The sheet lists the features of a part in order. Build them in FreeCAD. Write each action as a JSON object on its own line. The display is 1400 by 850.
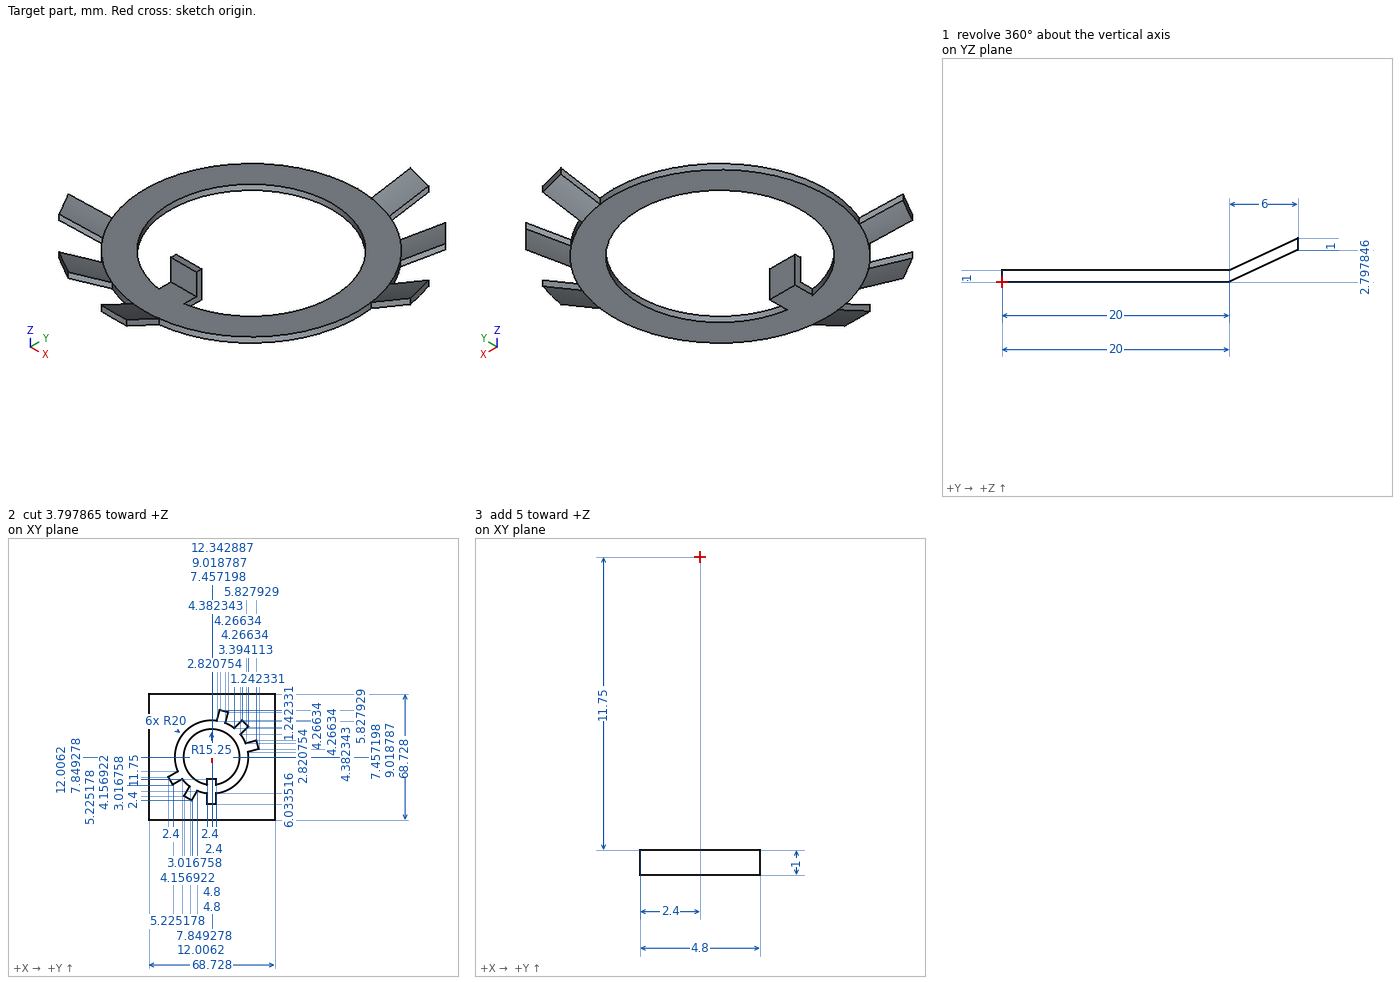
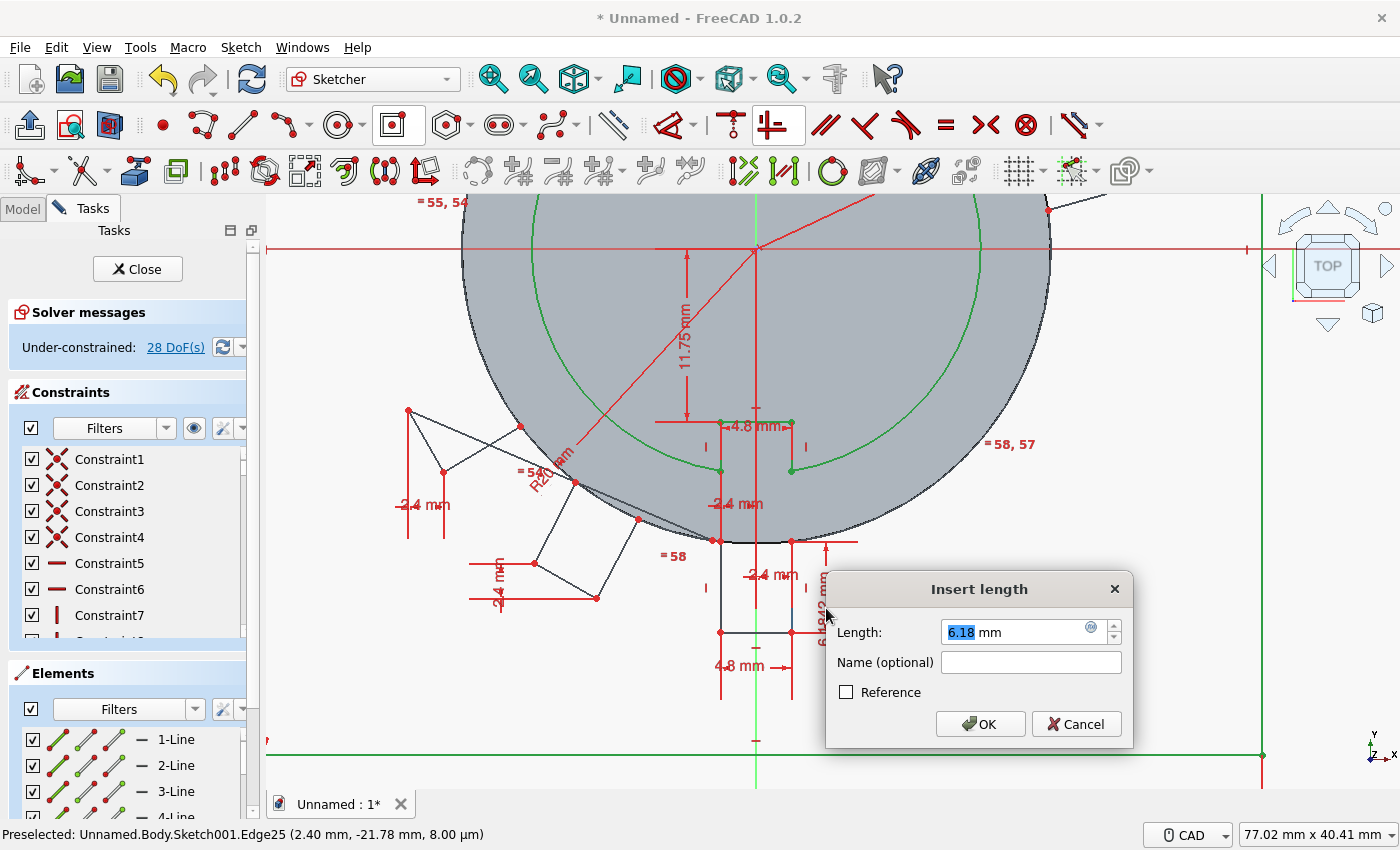
{"action": "type", "text": "6.033516"}
{"action": "key", "text": "Return"}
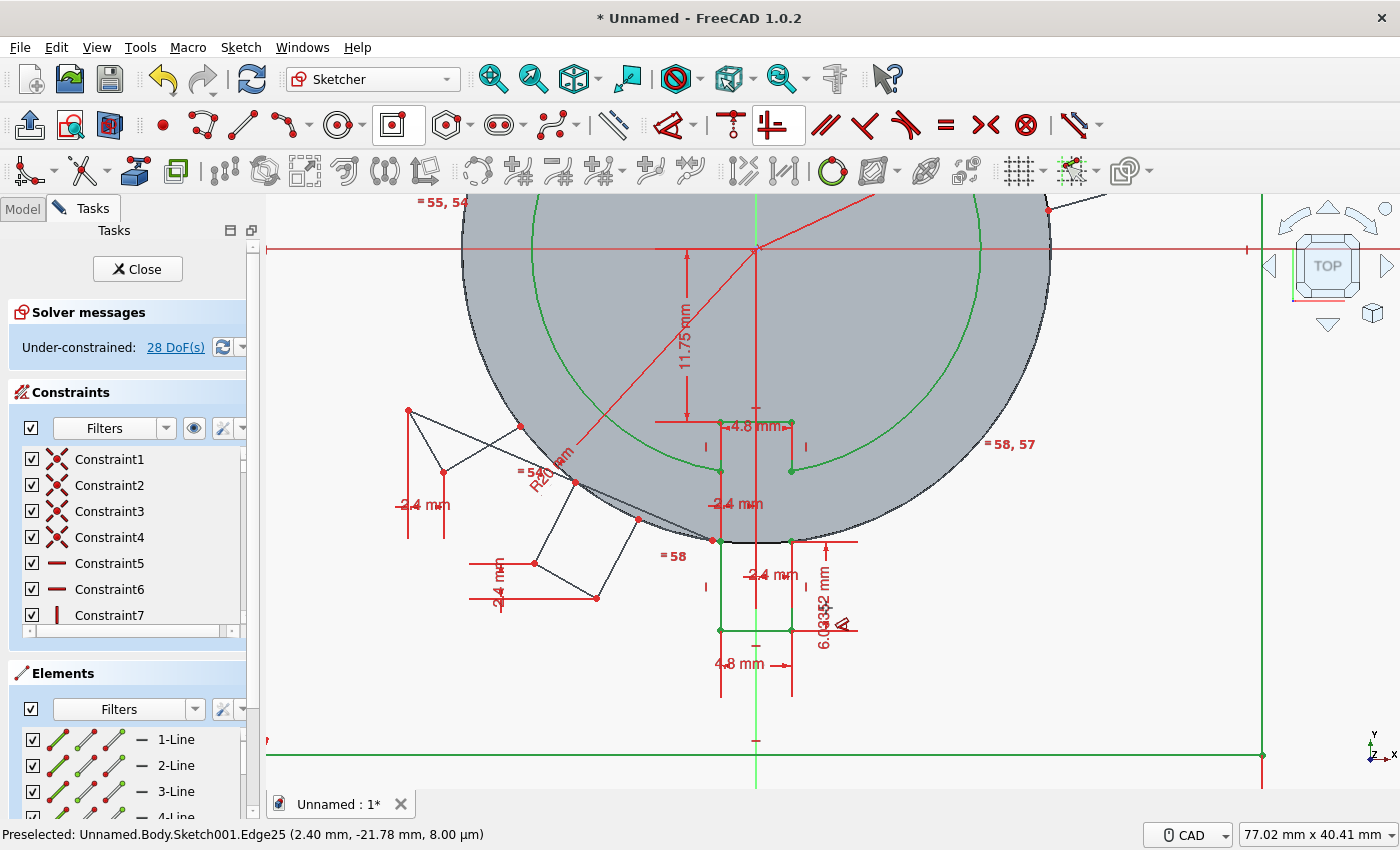
{"action": "left_click", "coordinate": [576, 482]}
{"action": "left_click", "coordinate": [603, 516]}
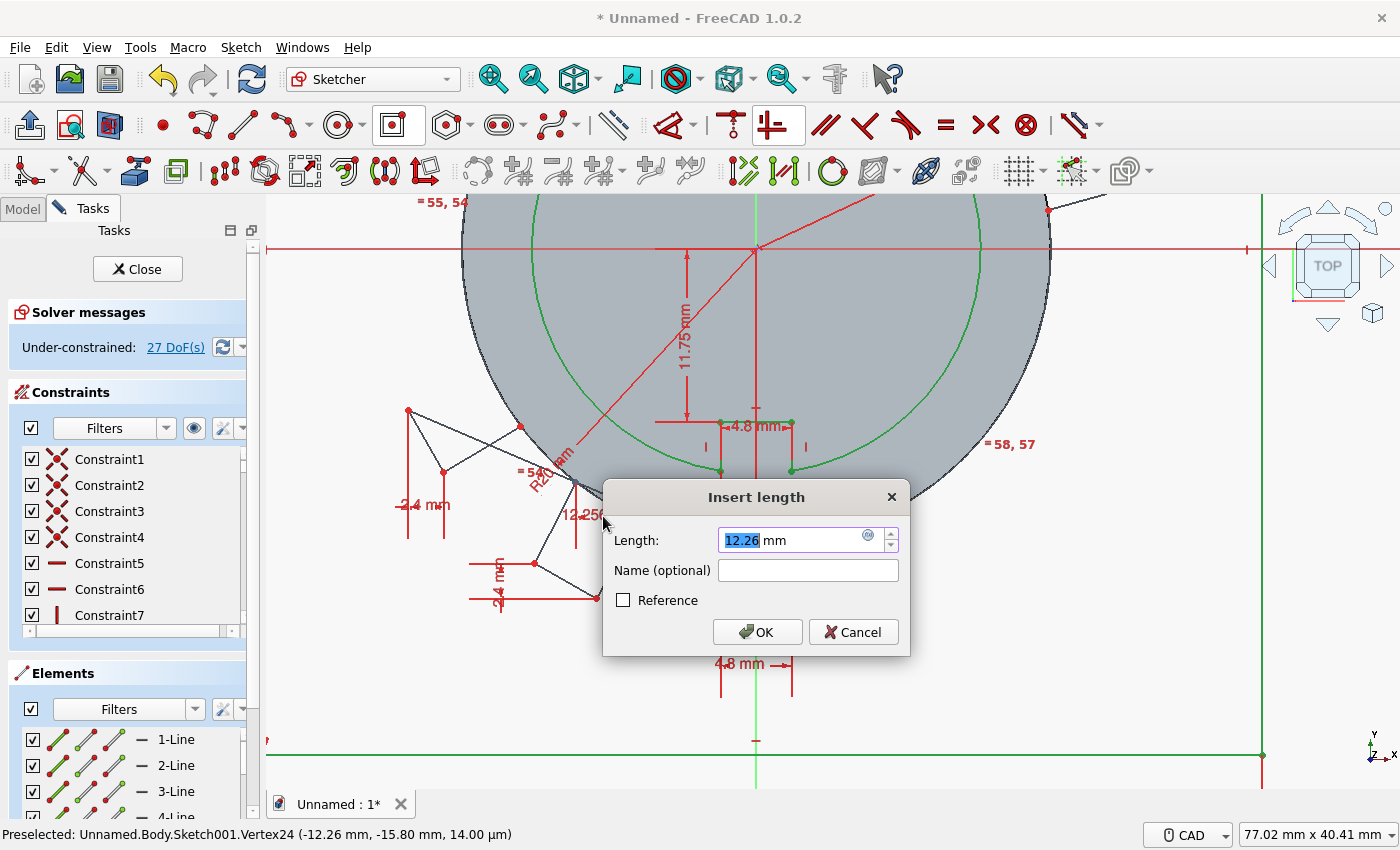
{"action": "type", "text": "12.0062"}
{"action": "key", "text": "Return"}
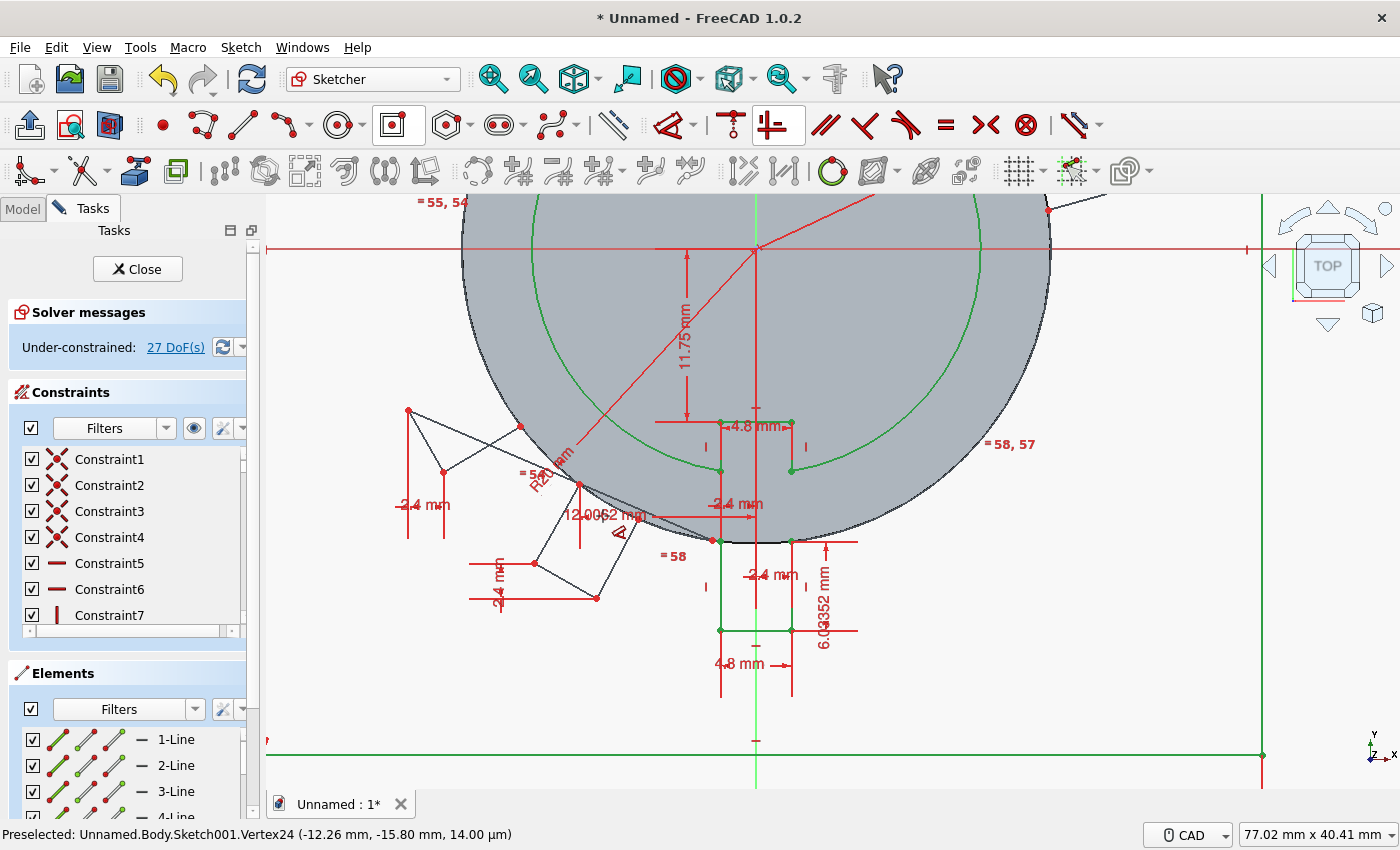
{"action": "left_click", "coordinate": [521, 426]}
{"action": "left_click", "coordinate": [487, 297]}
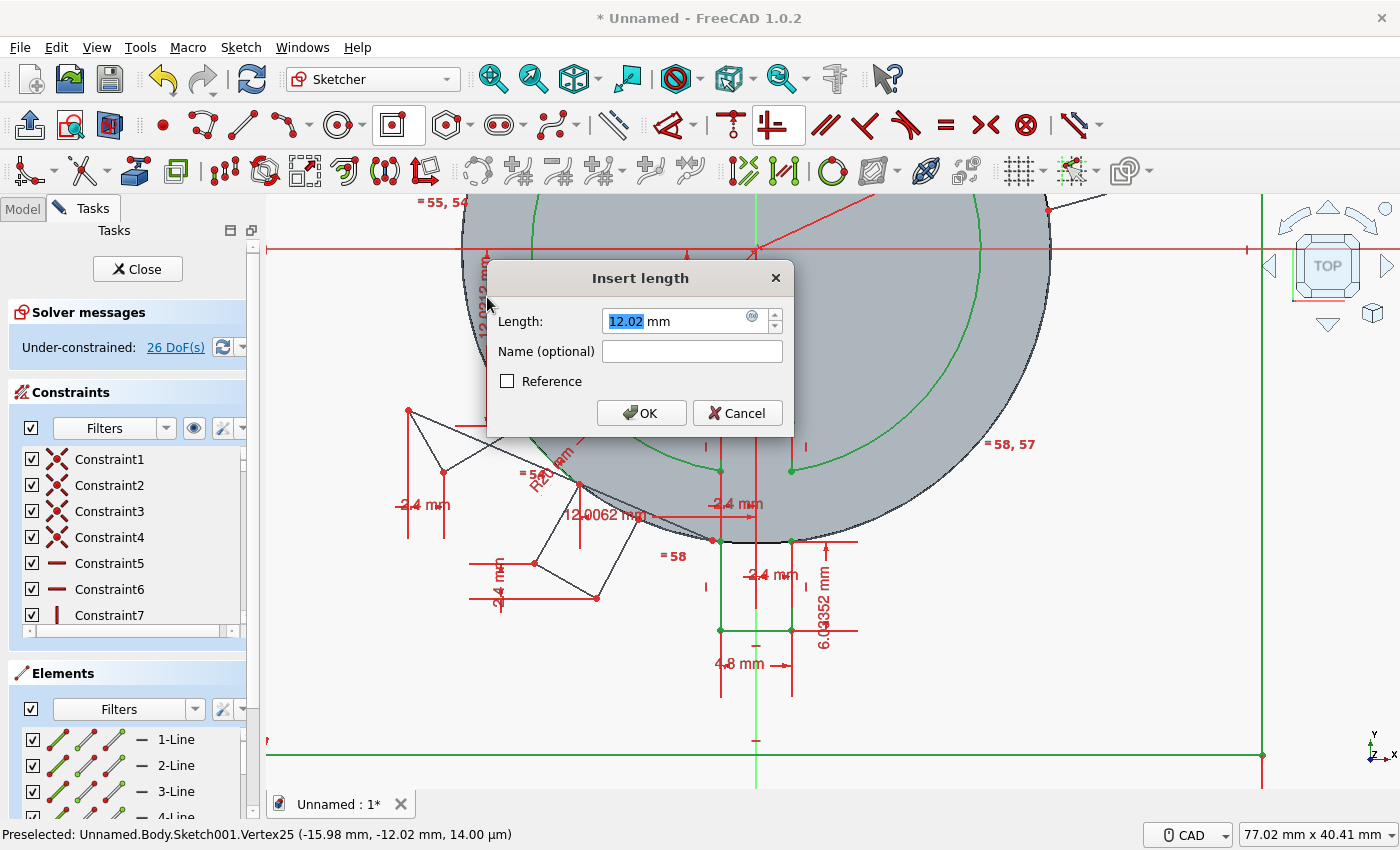
{"action": "type", "text": "12.0062"}
{"action": "key", "text": "Return"}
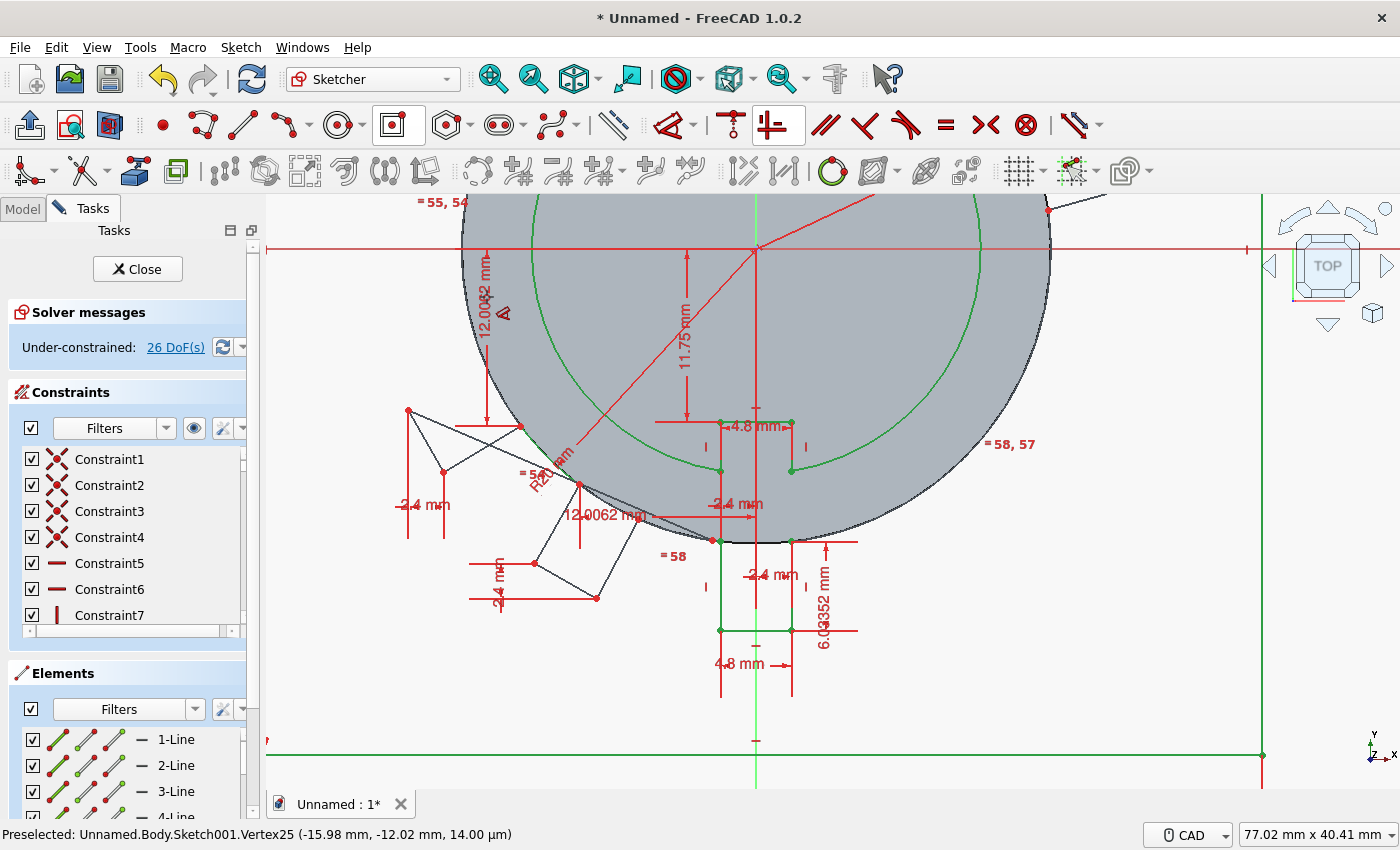
{"action": "scroll", "coordinate": [769, 632], "scroll_direction": "down", "scroll_amount": 5}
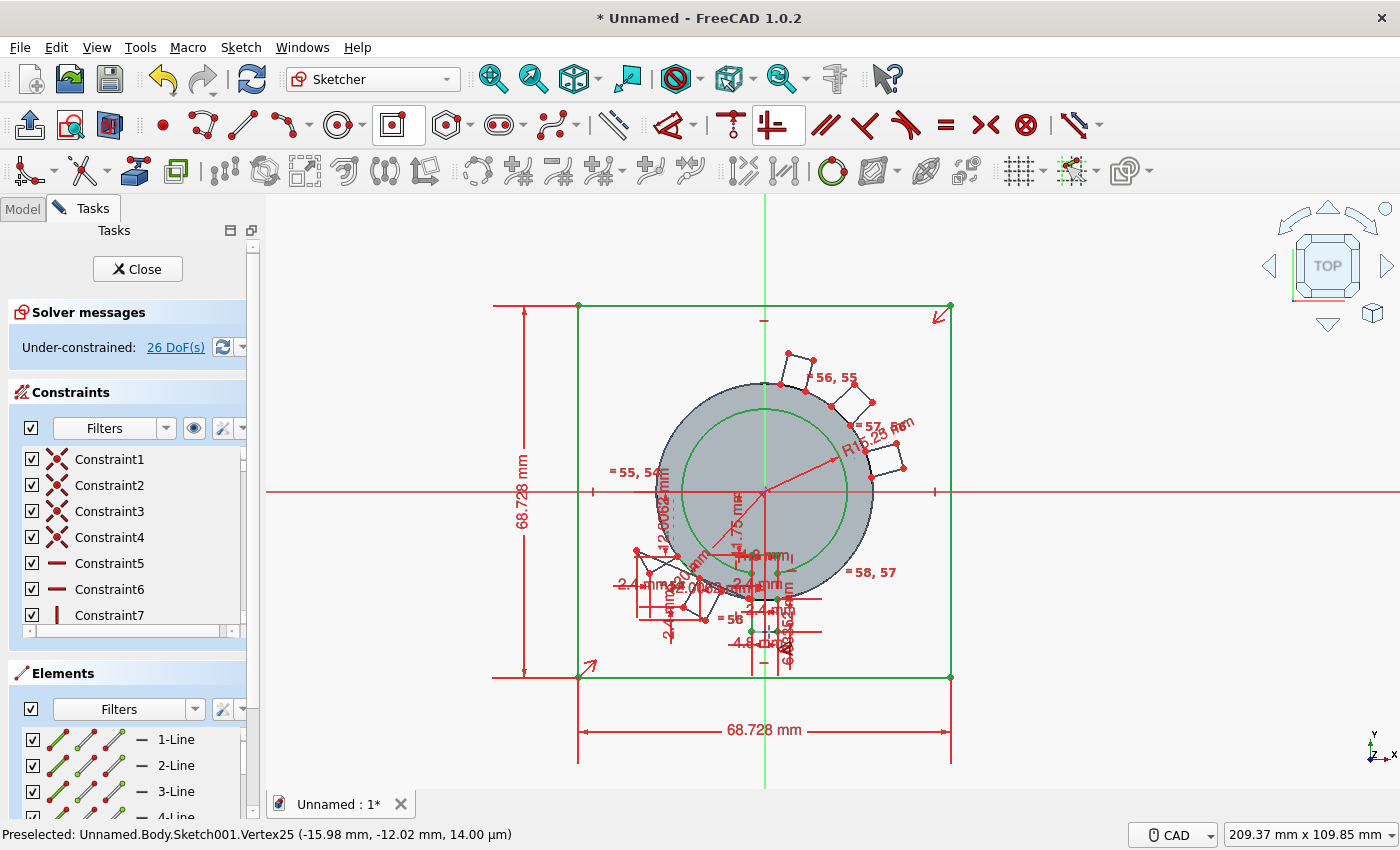
{"action": "scroll", "coordinate": [838, 400], "scroll_direction": "up", "scroll_amount": 3}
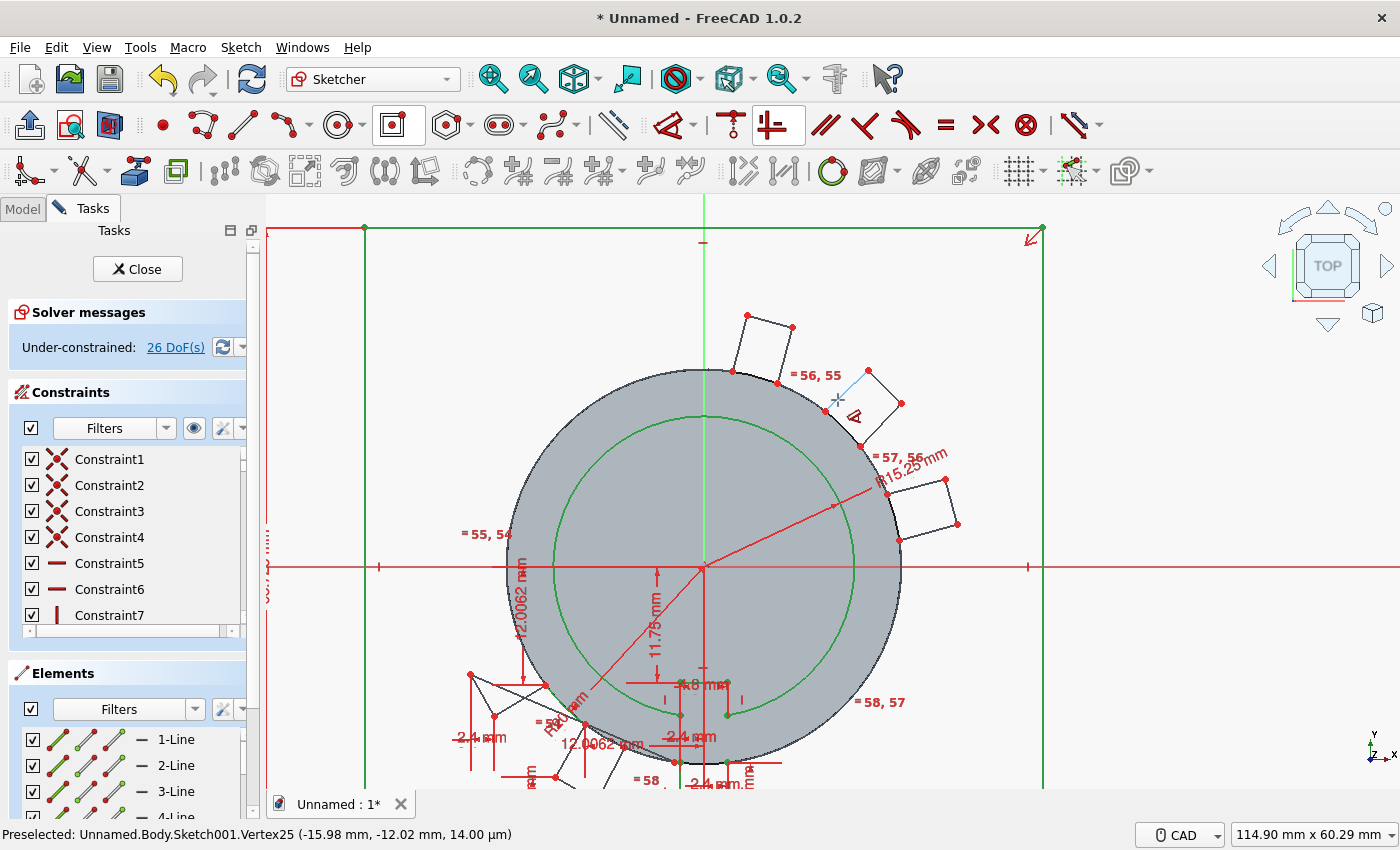
{"action": "left_click", "coordinate": [838, 399]}
{"action": "left_click", "coordinate": [847, 337]}